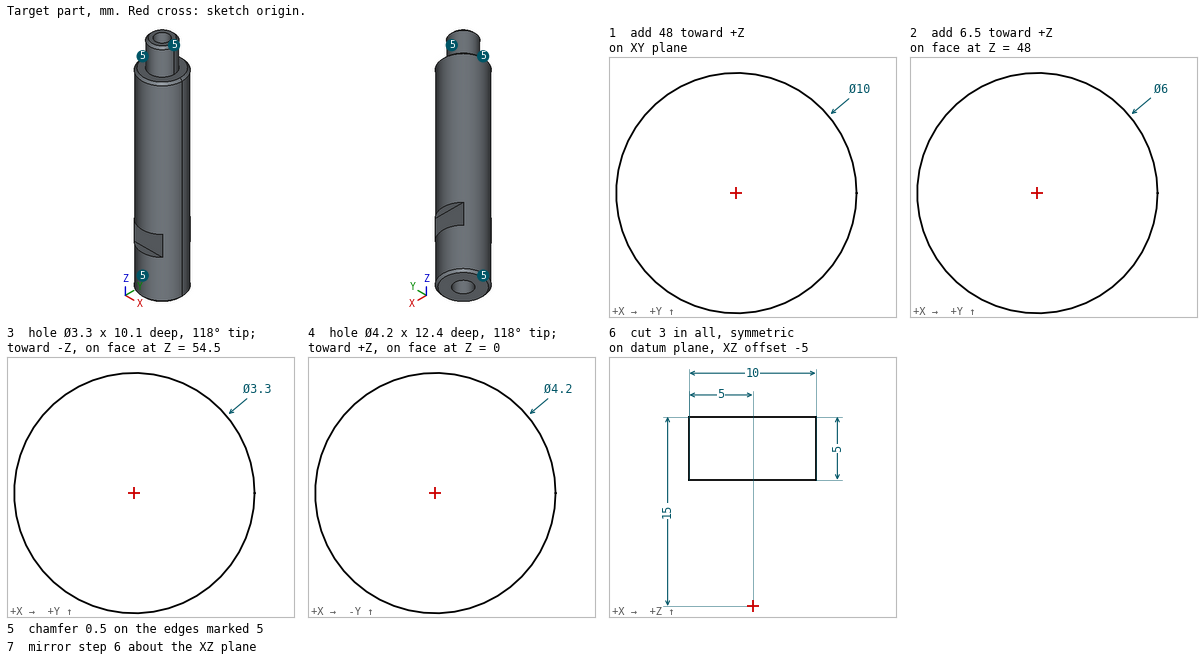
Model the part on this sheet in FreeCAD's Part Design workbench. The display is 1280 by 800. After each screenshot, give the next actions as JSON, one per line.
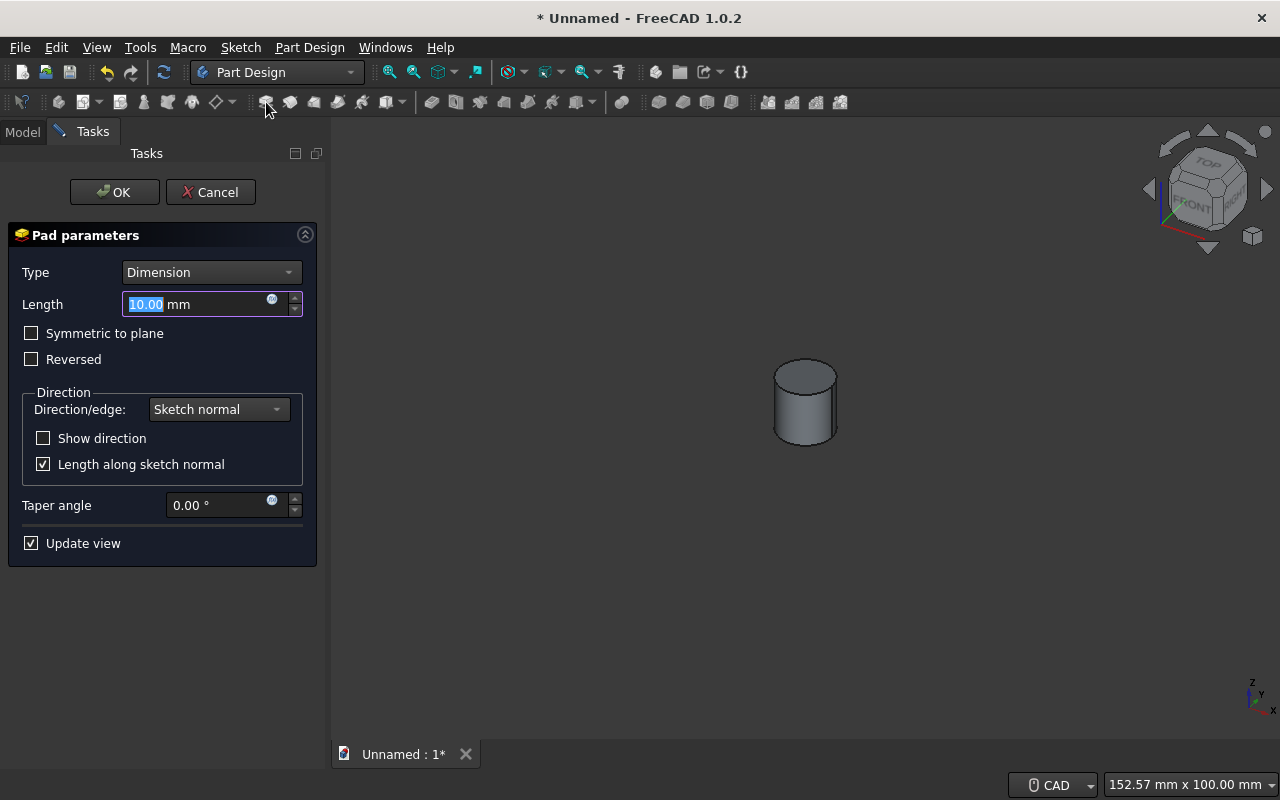
{"action": "type", "text": "48"}
{"action": "key", "text": "Tab"}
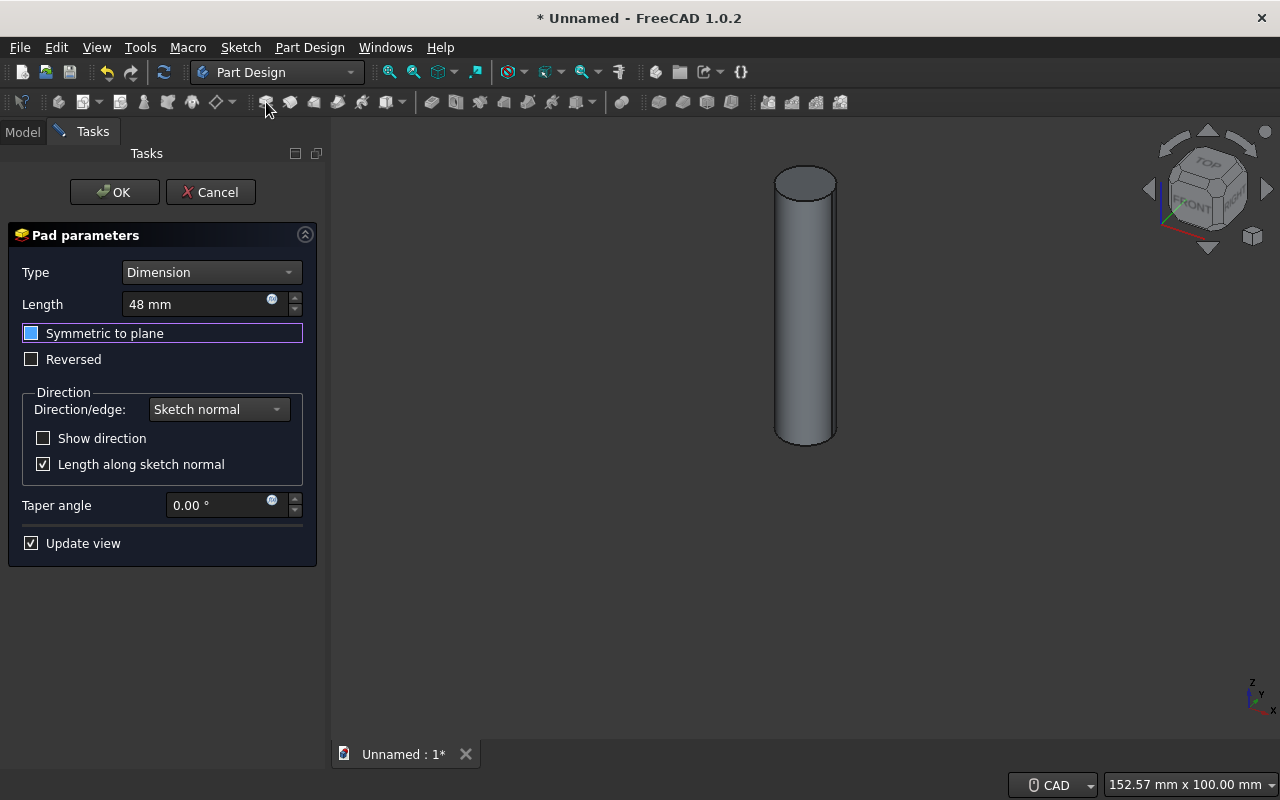
{"action": "left_click", "coordinate": [115, 192]}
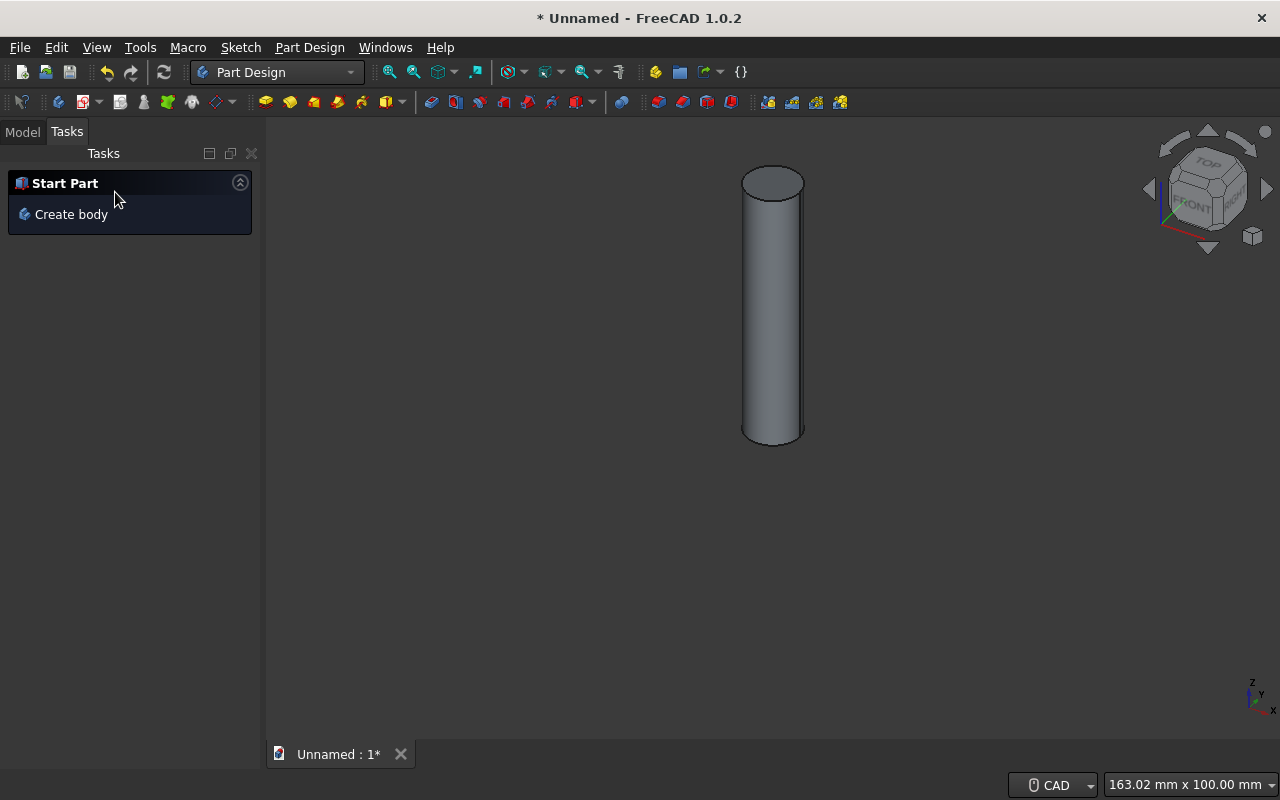
{"action": "left_click", "coordinate": [773, 182]}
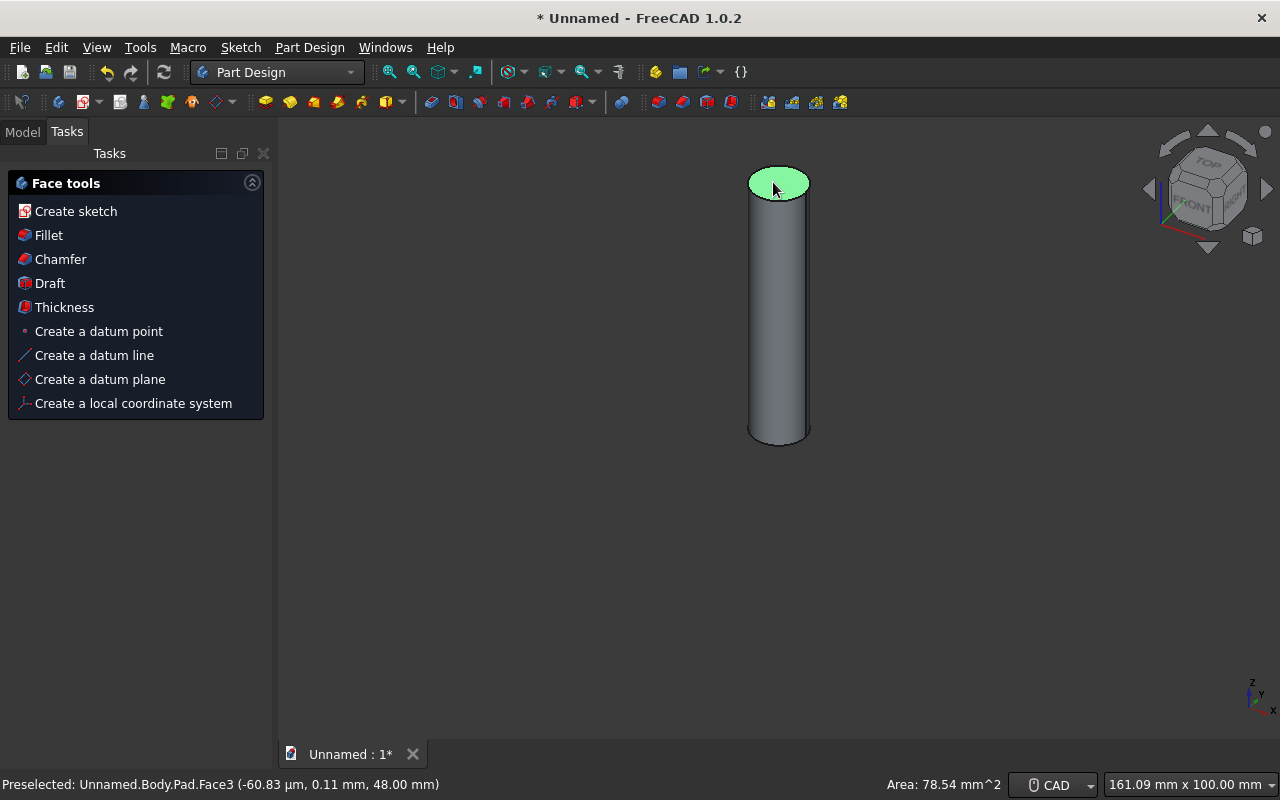
{"action": "left_click", "coordinate": [84, 102]}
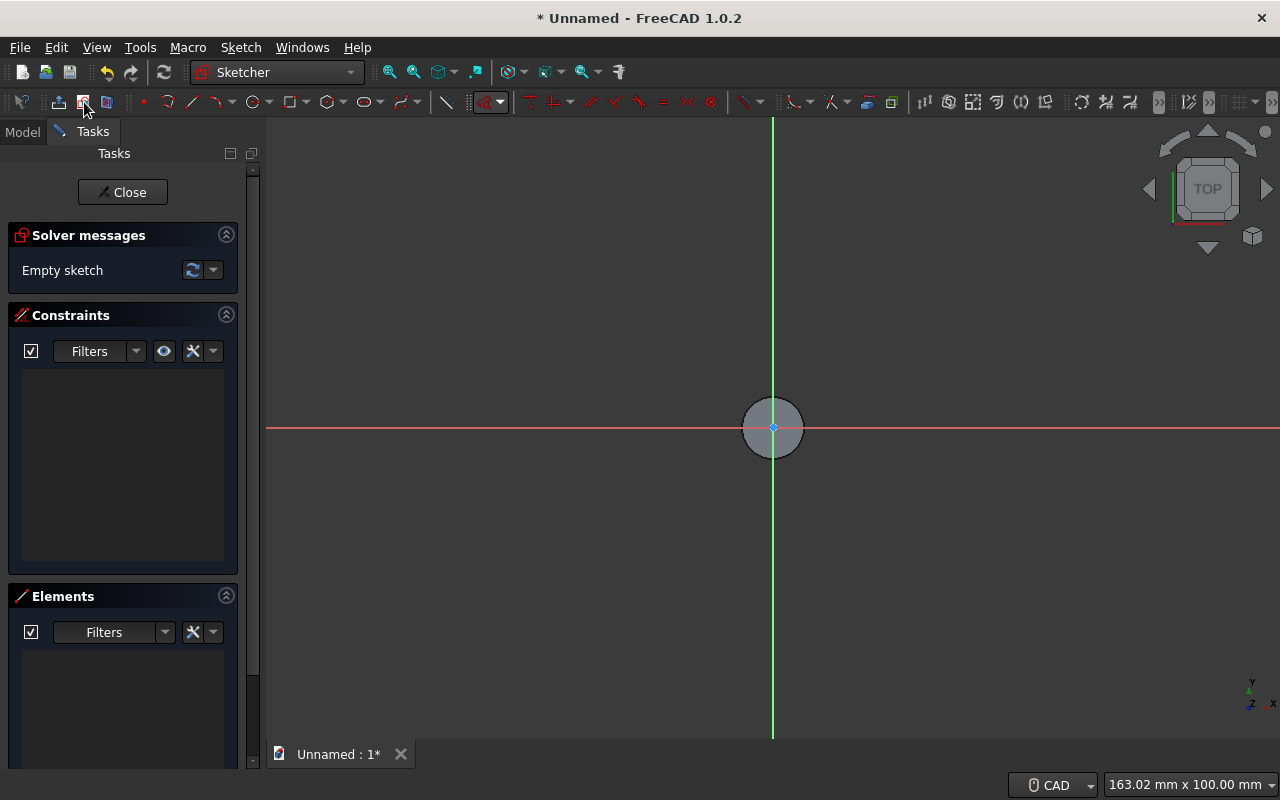
{"action": "scroll", "coordinate": [780, 428], "scroll_direction": "up", "scroll_amount": 12}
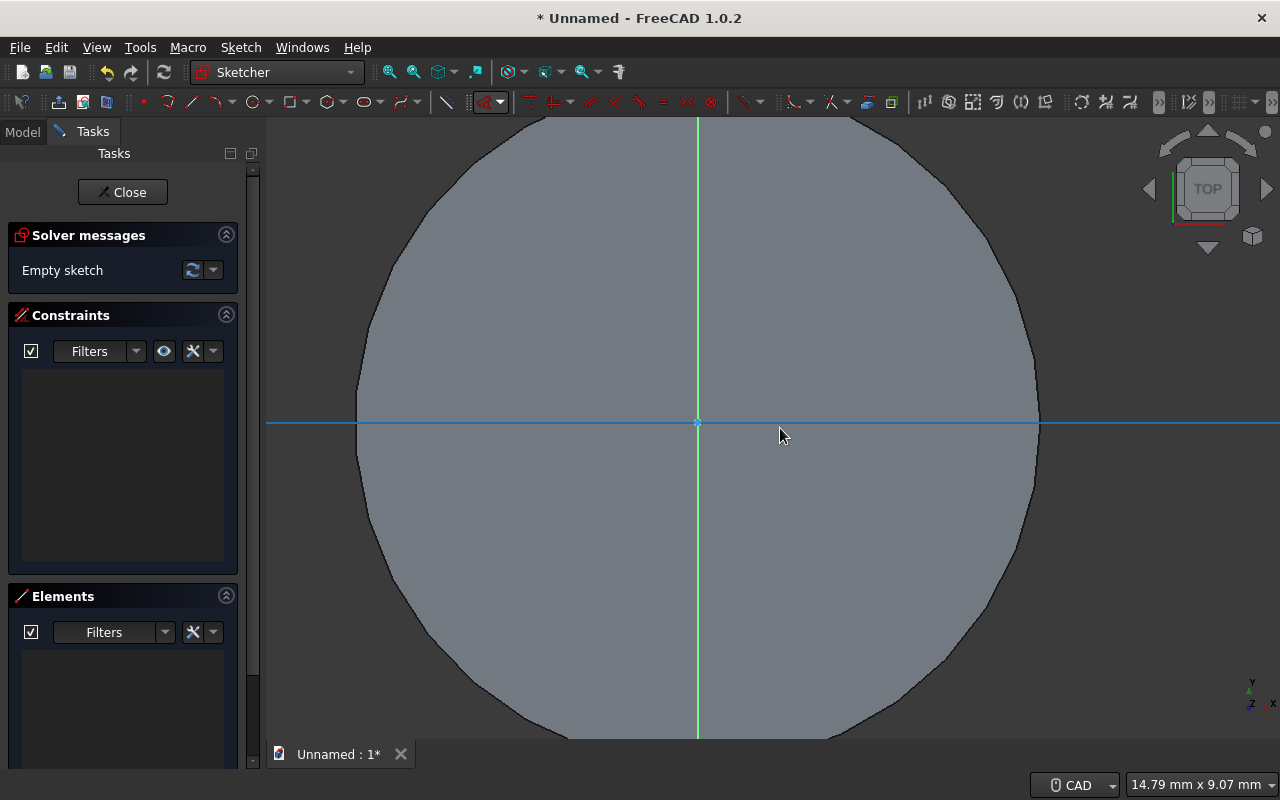
{"action": "key", "text": "g c"}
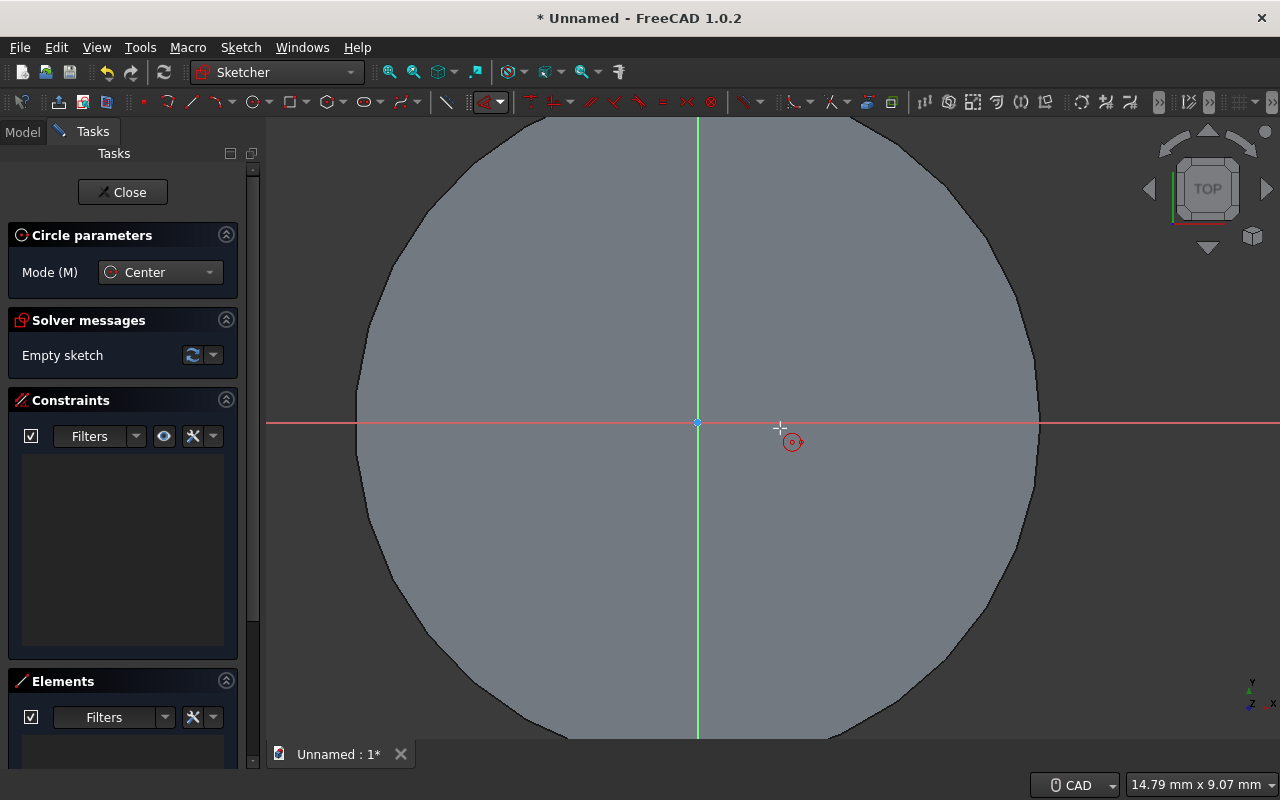
{"action": "left_click", "coordinate": [698, 423]}
{"action": "mouse_move", "coordinate": [843, 278]}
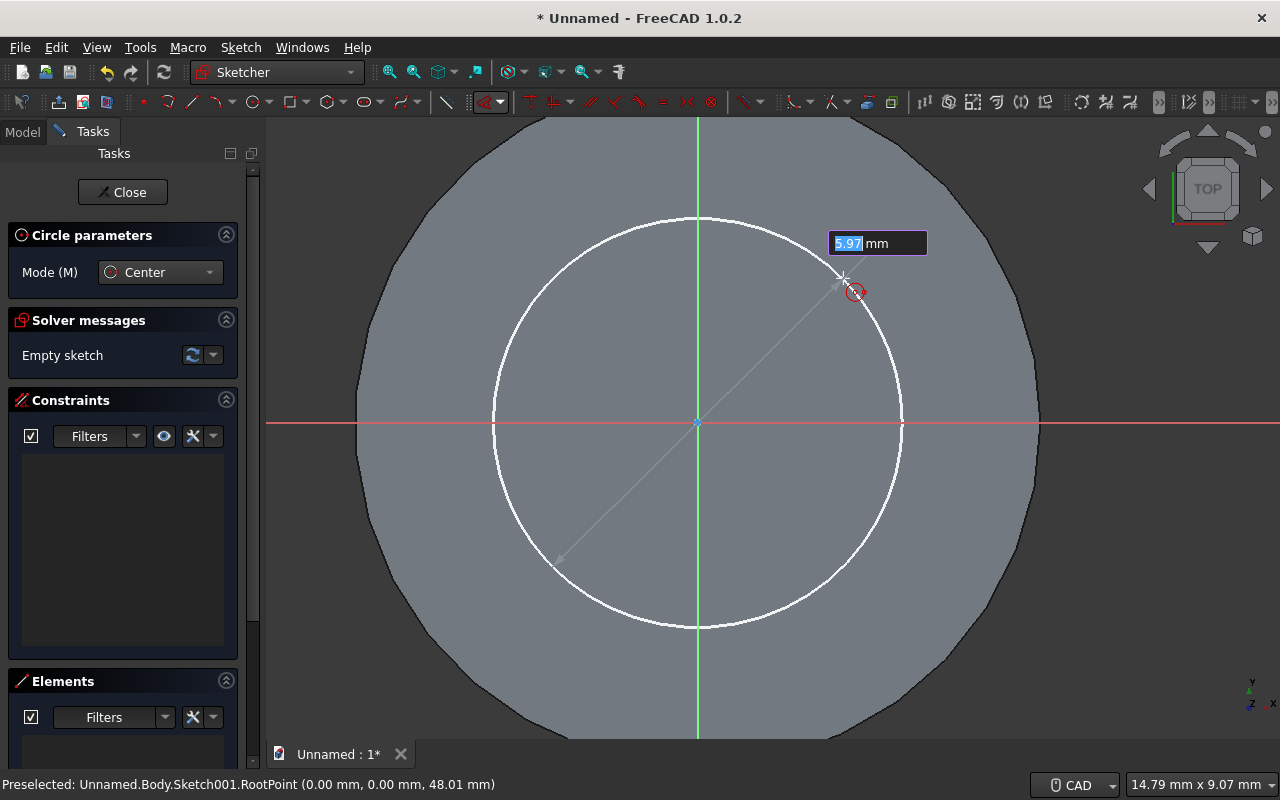
{"action": "type", "text": "6"}
{"action": "key", "text": "Return"}
{"action": "key", "text": "Escape"}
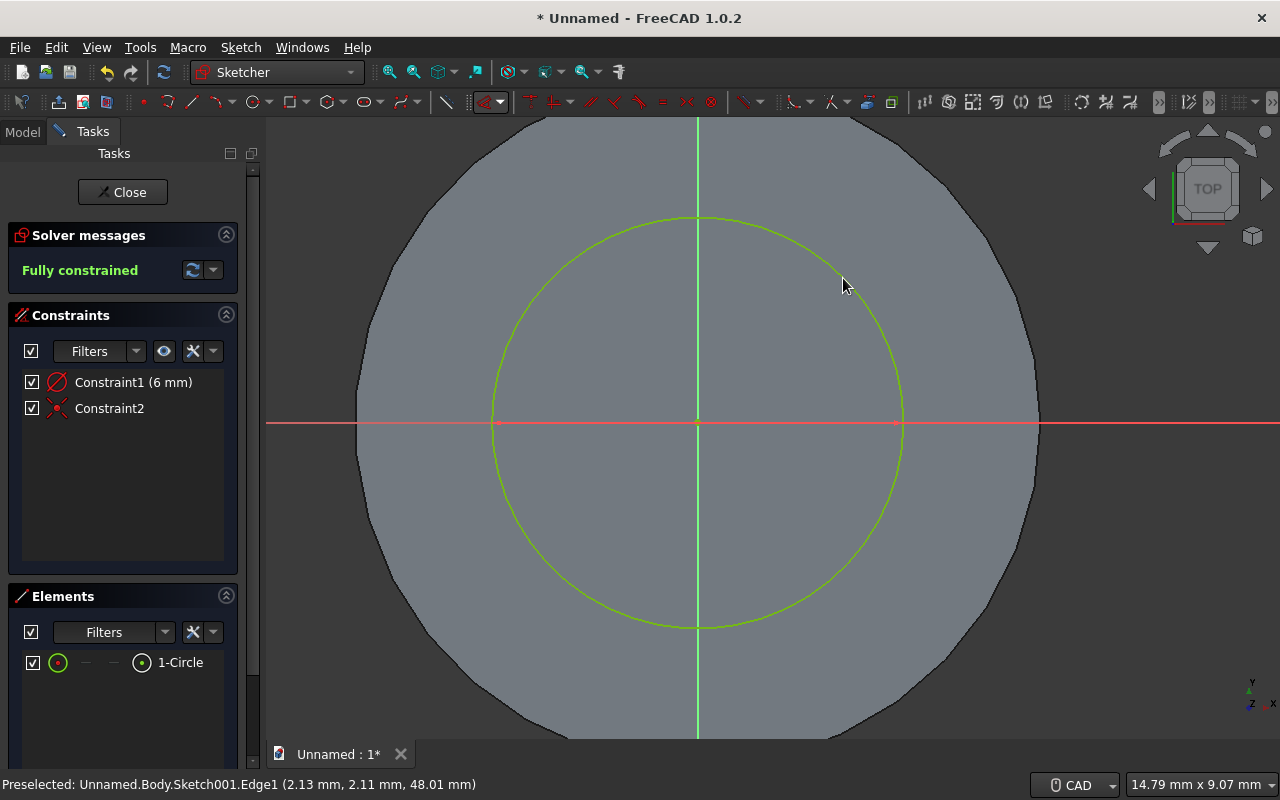
{"action": "left_click", "coordinate": [123, 192]}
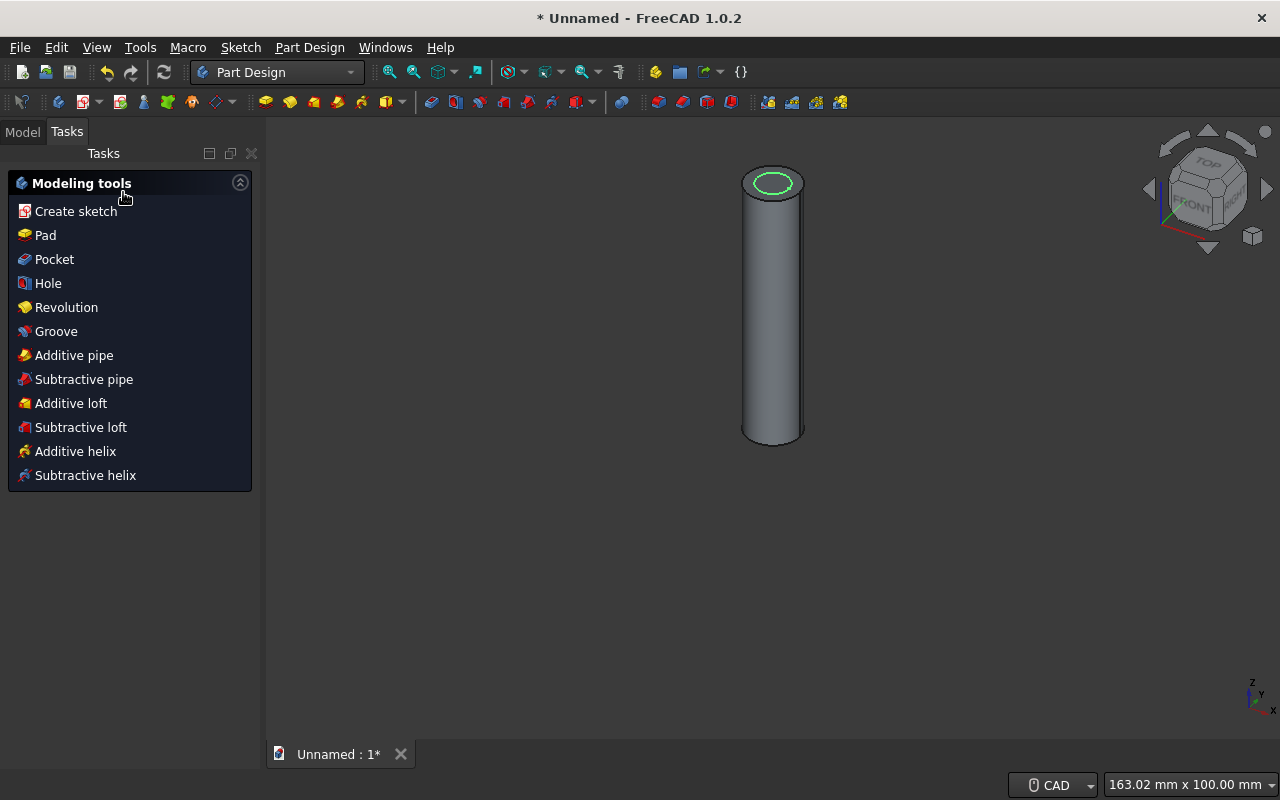
{"action": "left_click", "coordinate": [266, 102]}